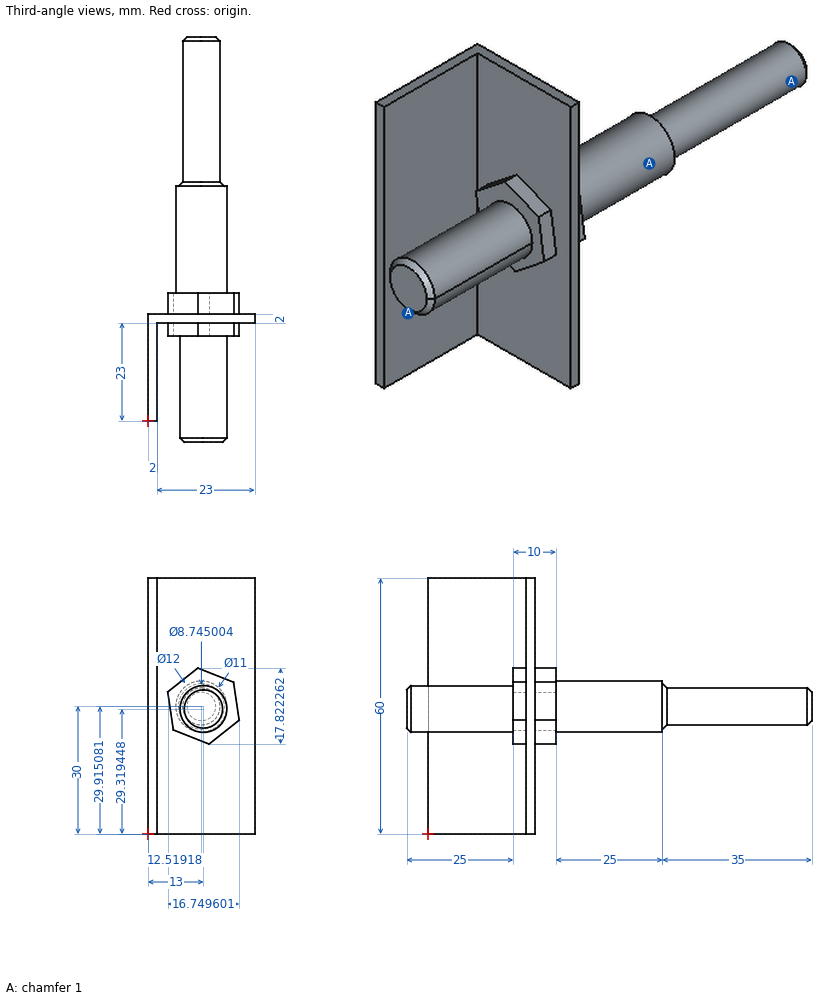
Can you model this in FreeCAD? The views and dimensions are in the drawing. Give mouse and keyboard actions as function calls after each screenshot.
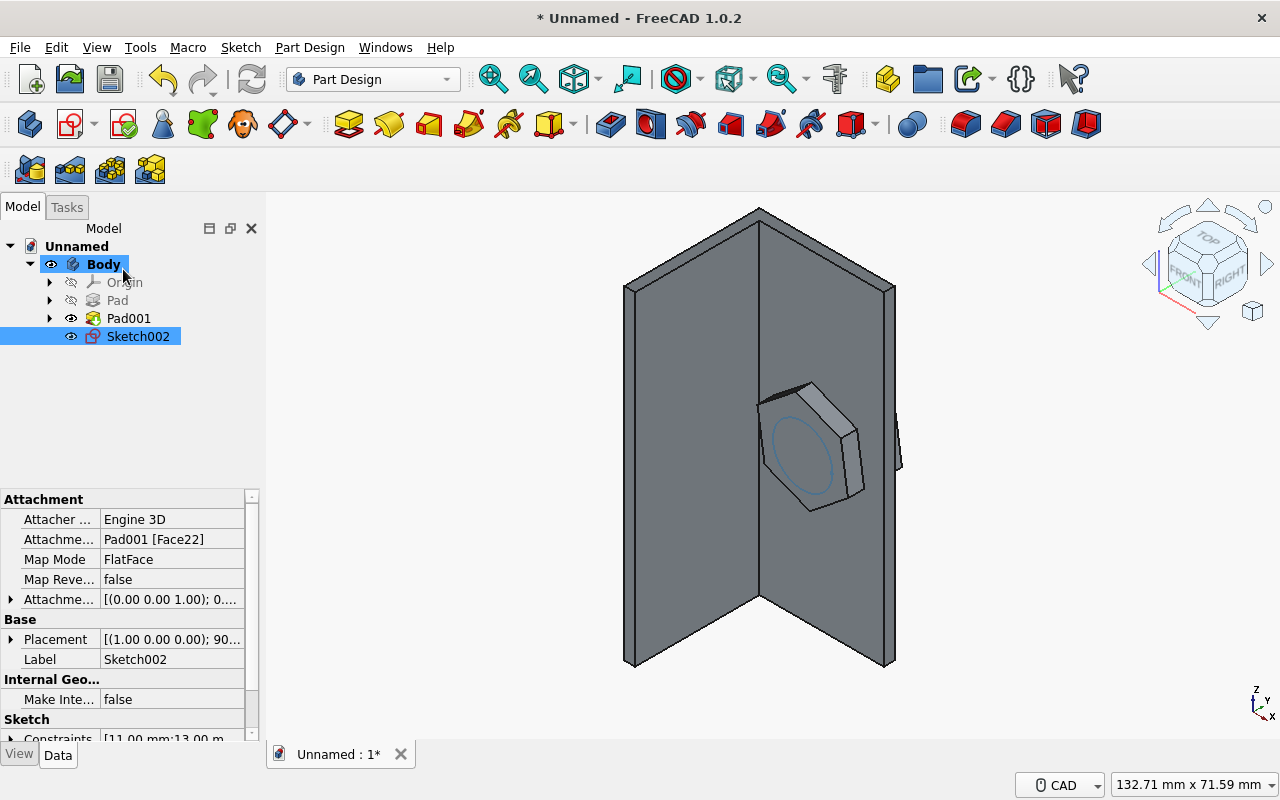
click(350, 124)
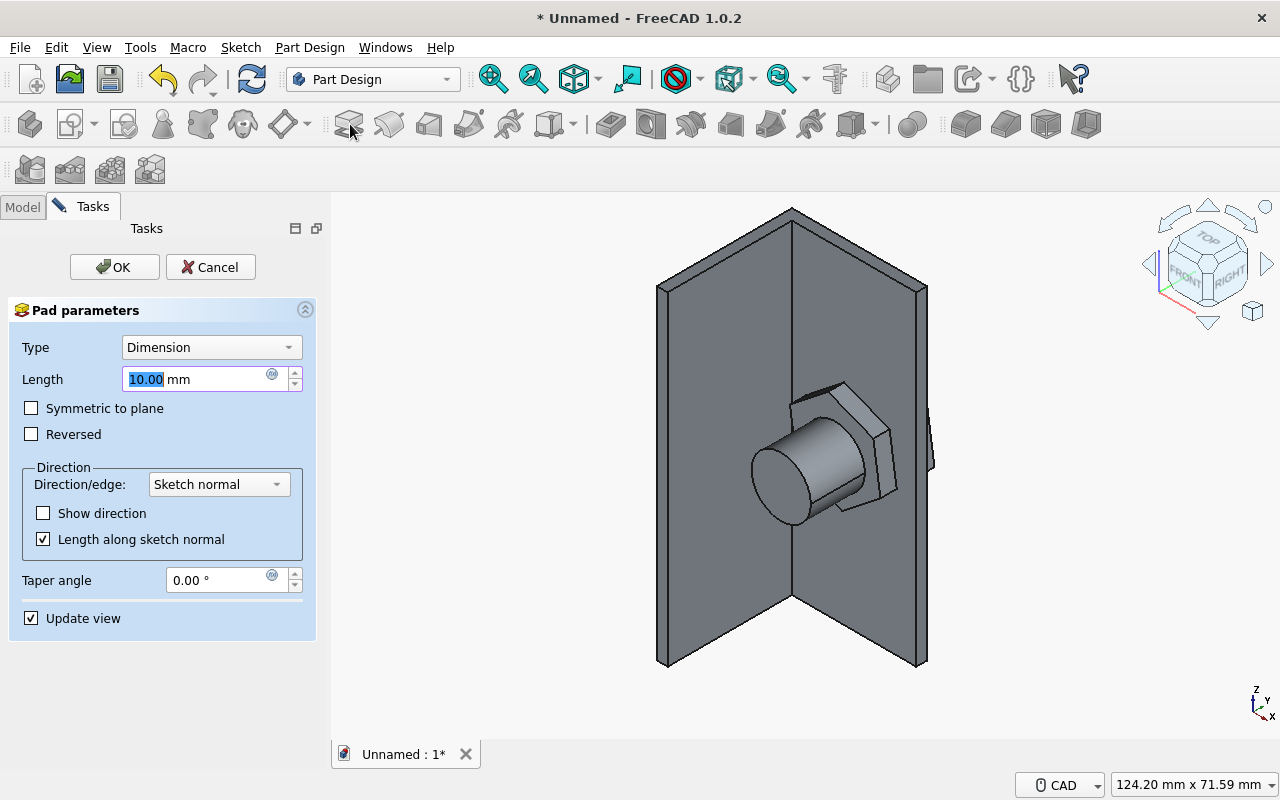
text(25)
key(Tab)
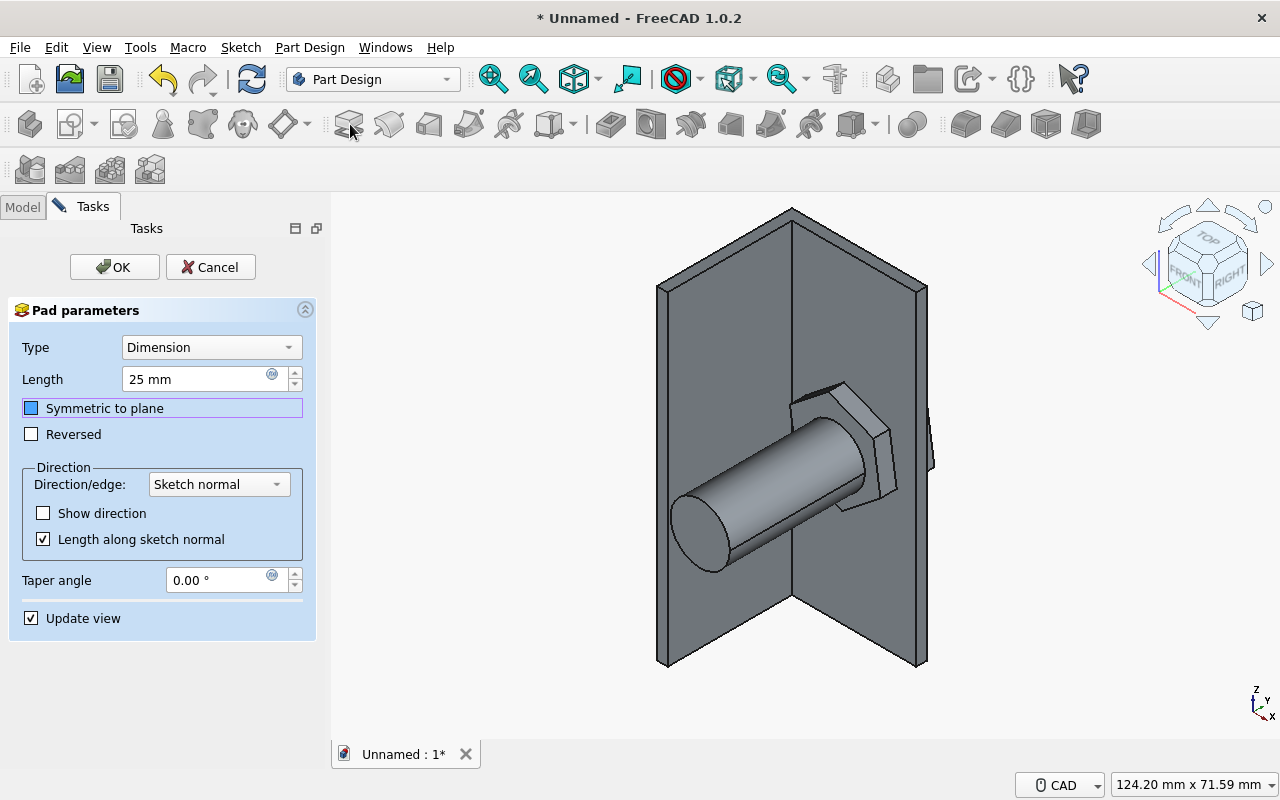
click(115, 267)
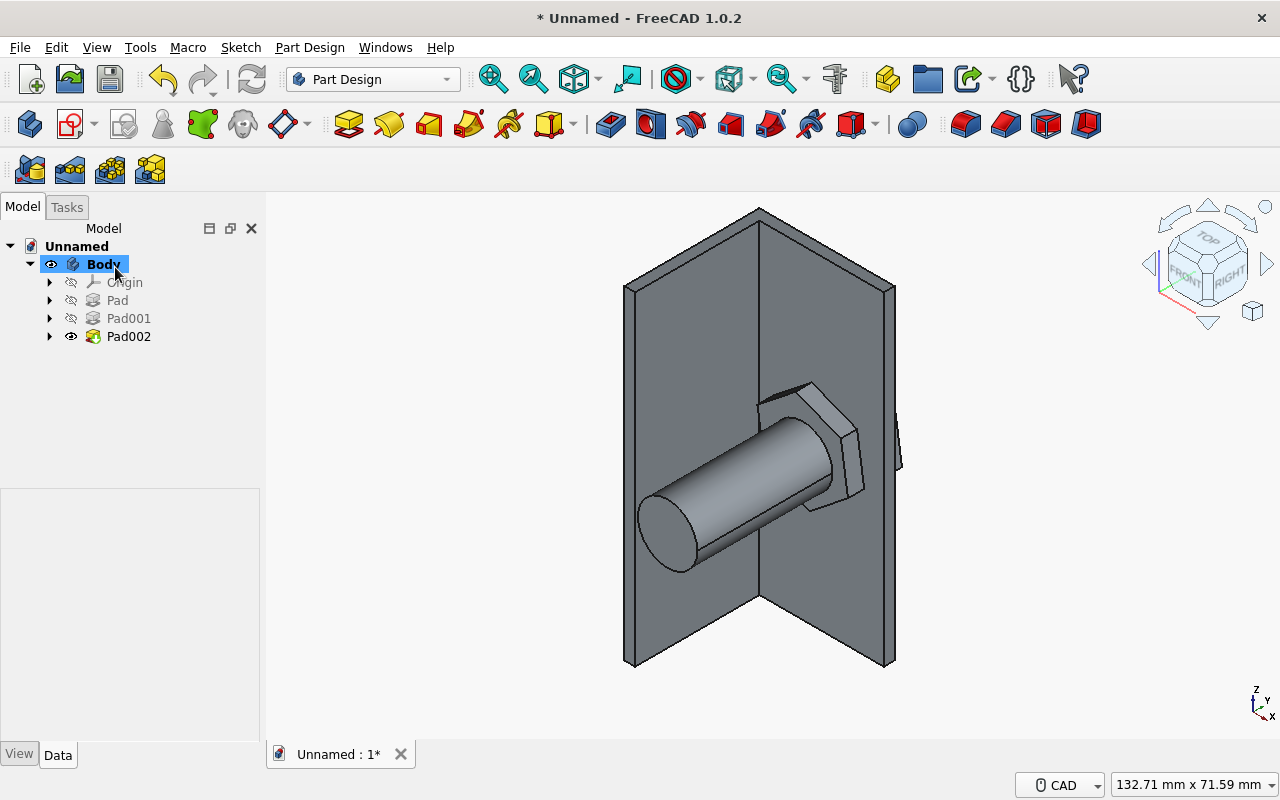
key(v)
key(f)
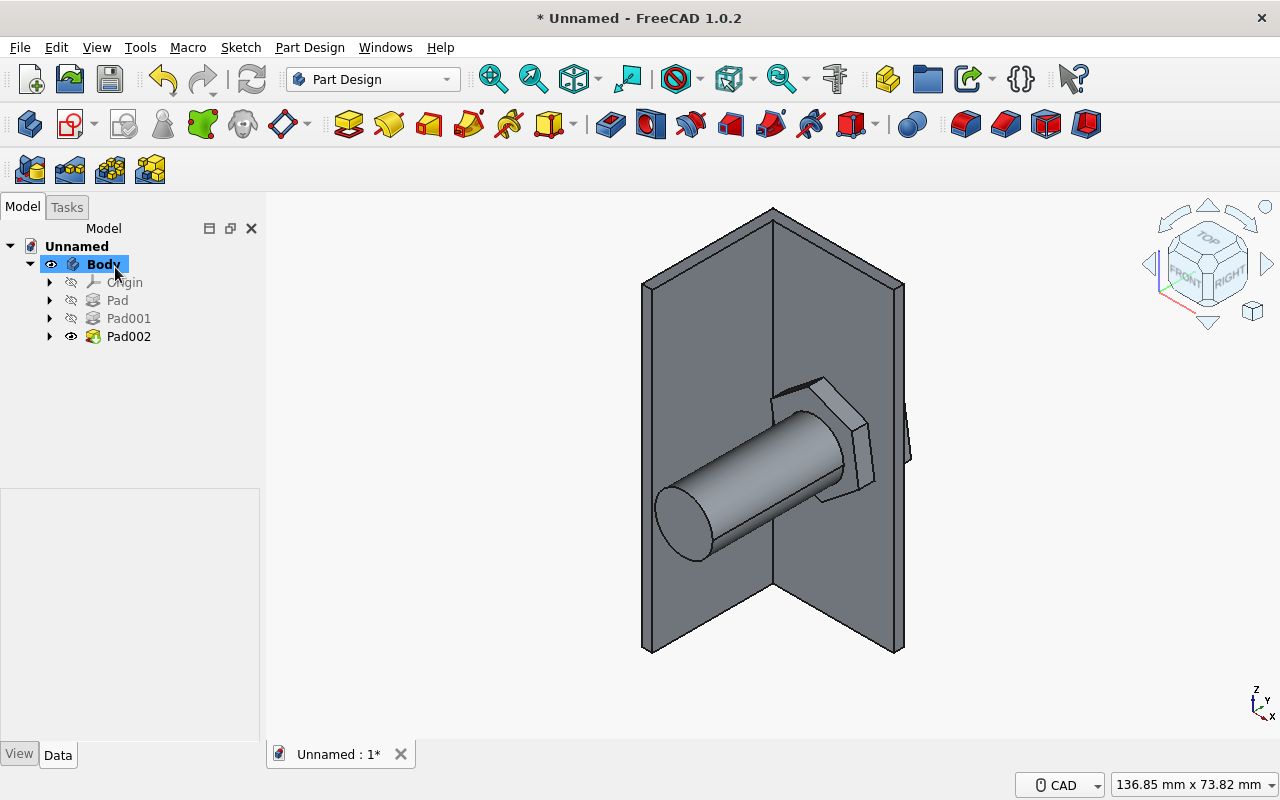
key(4)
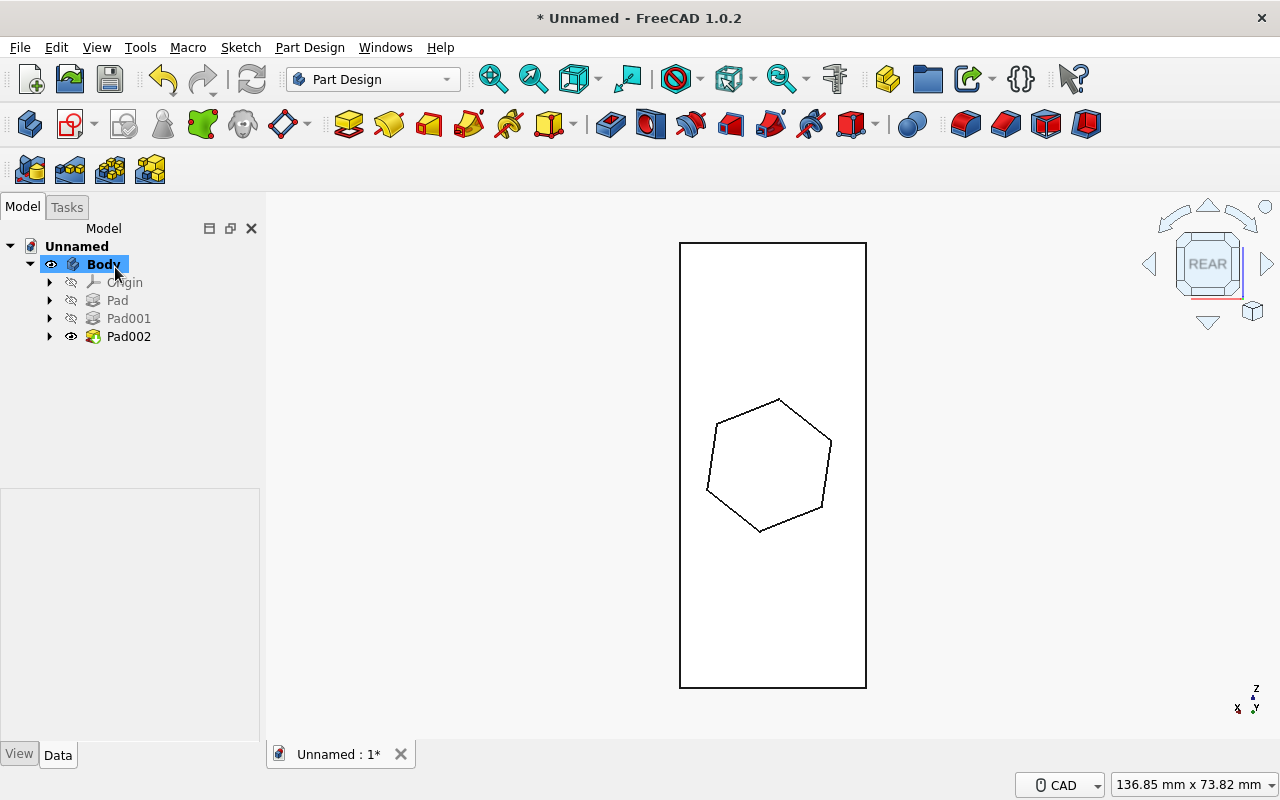
click(769, 465)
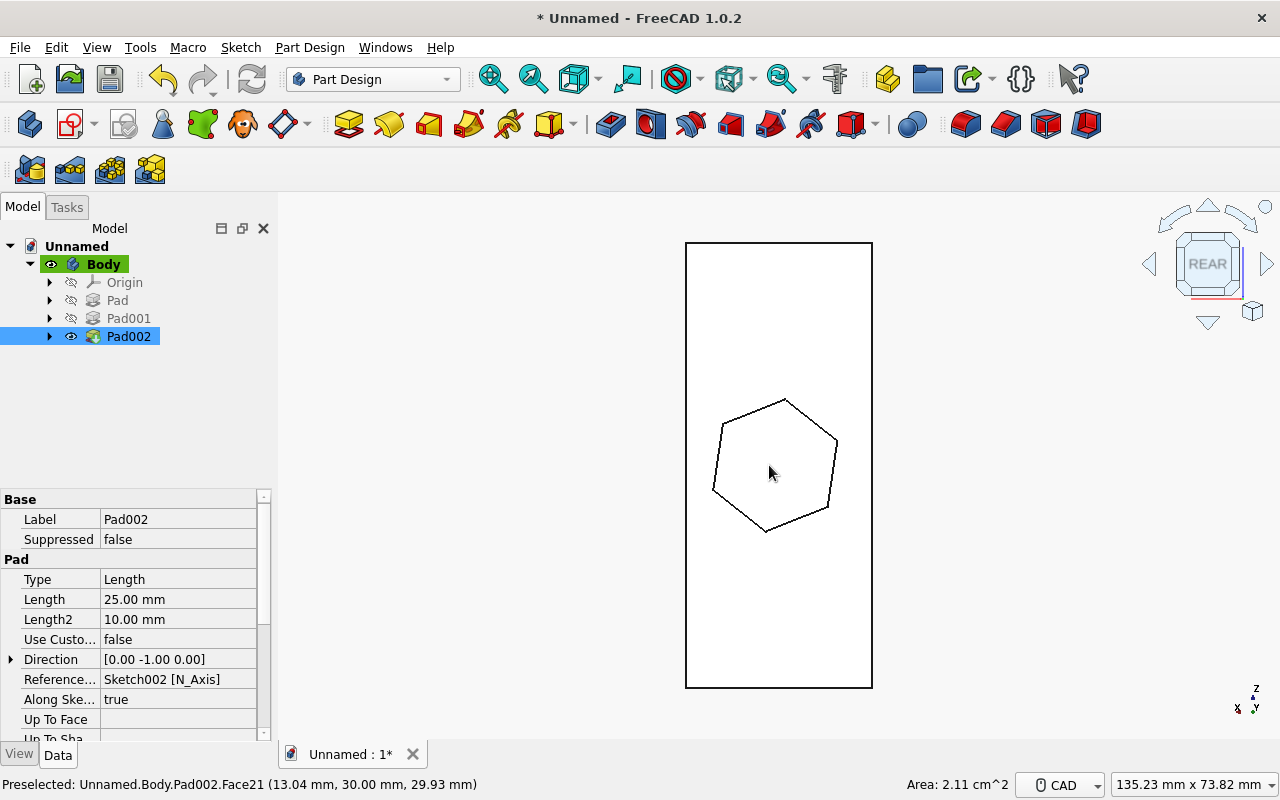
click(70, 124)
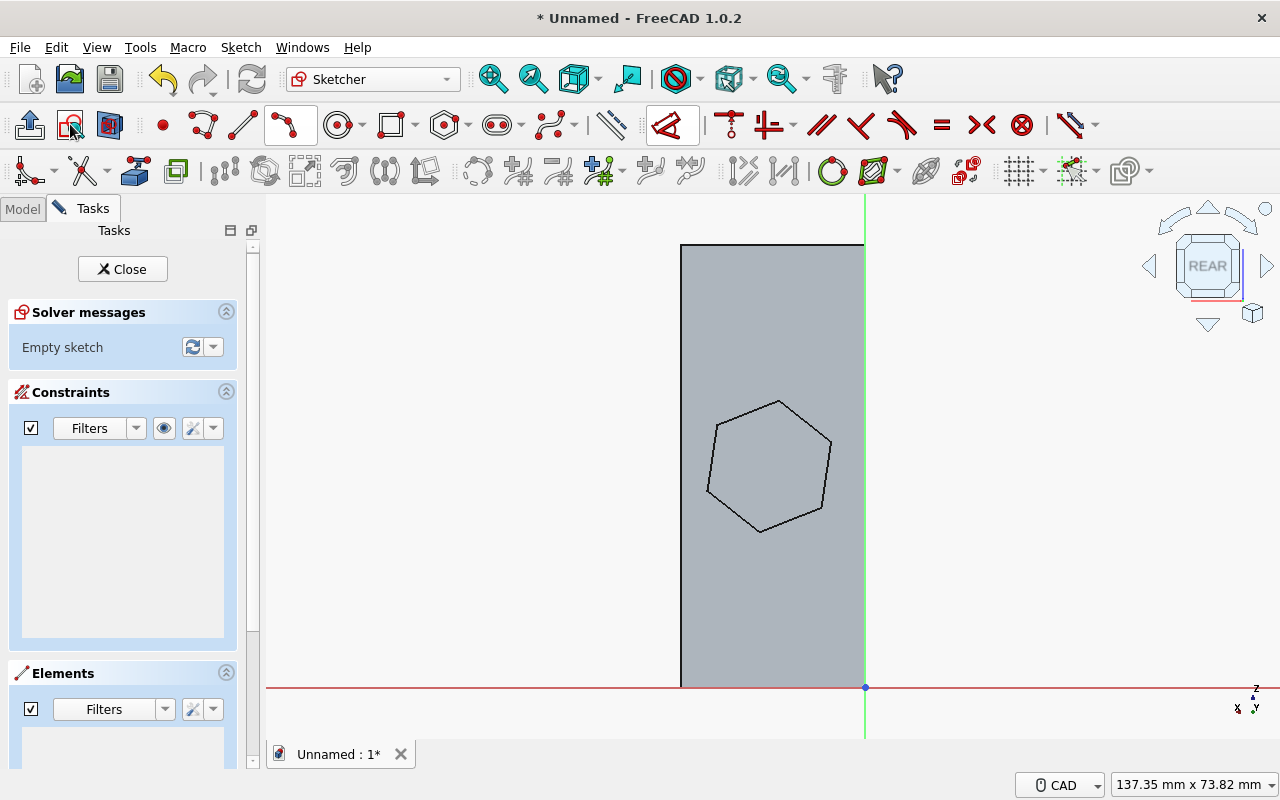
scroll(795, 467, up, 7)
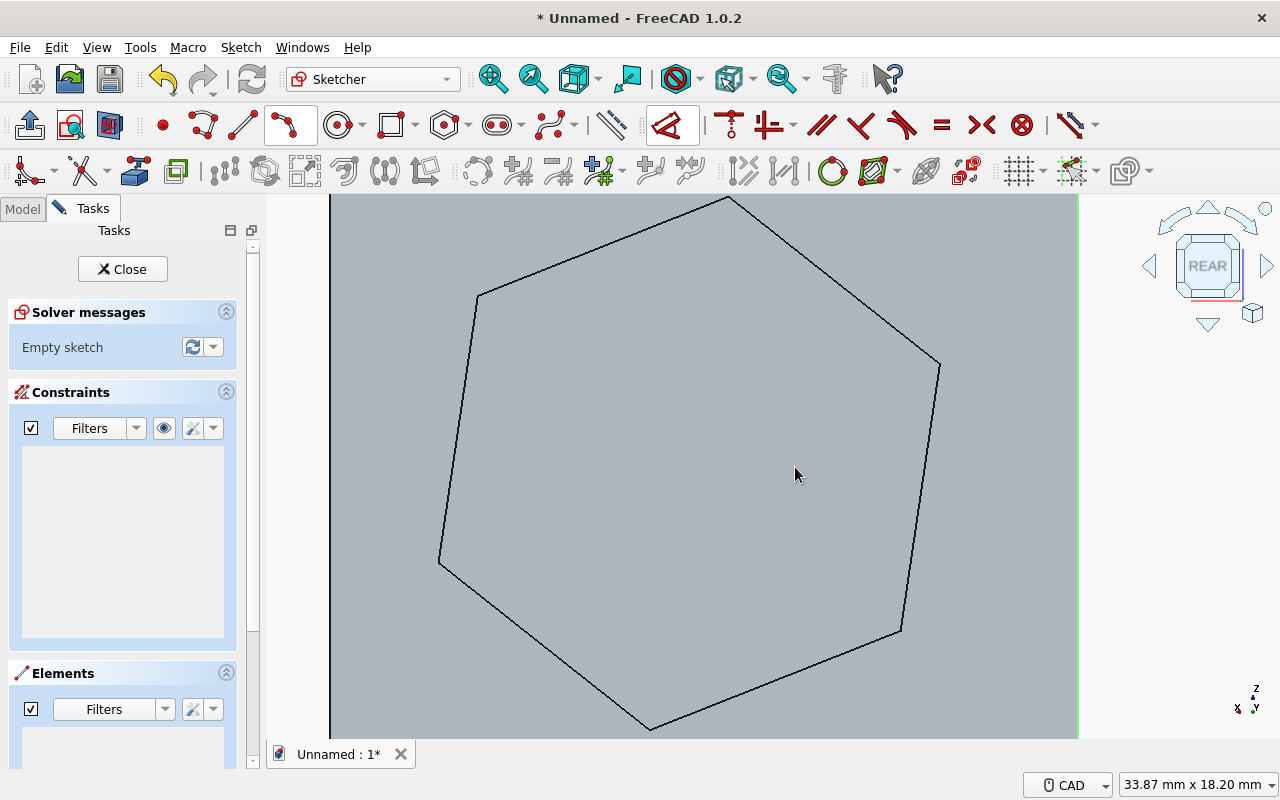
key(g)
key(c)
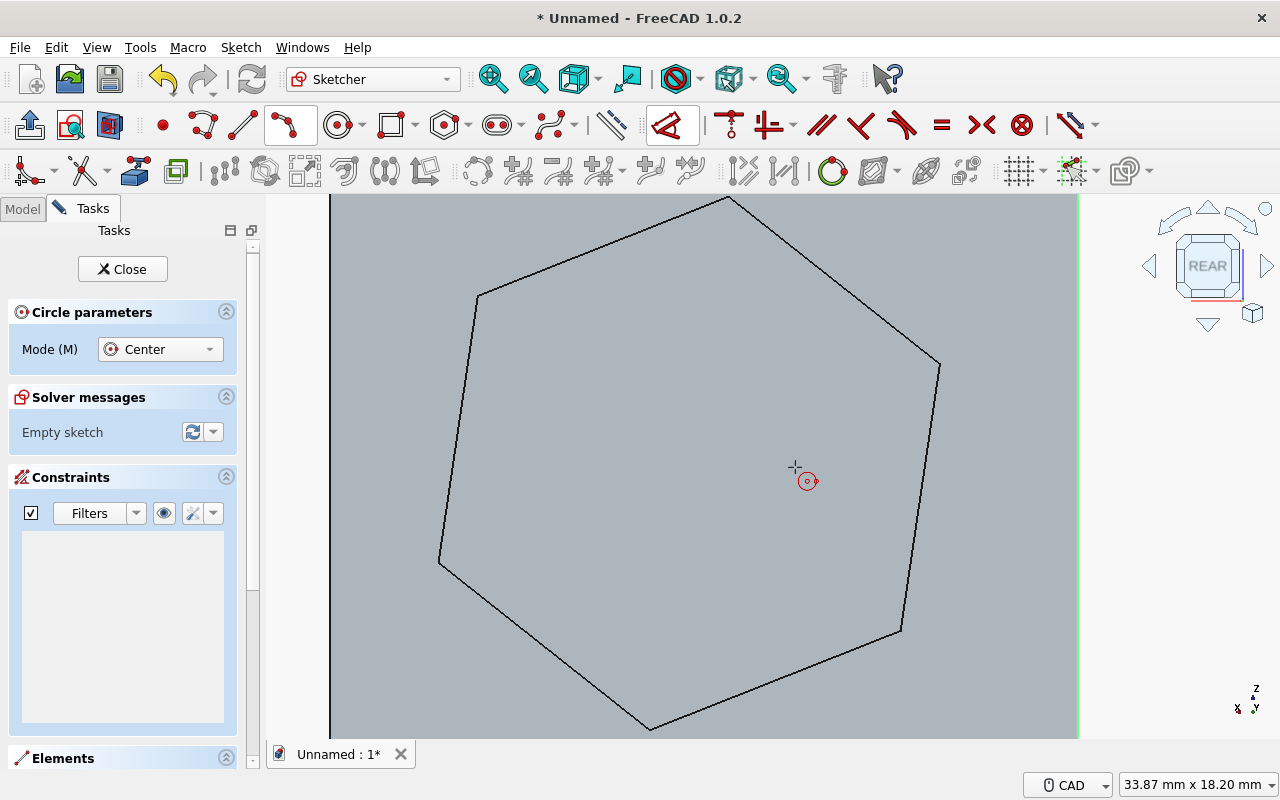
click(704, 466)
click(831, 339)
key(Escape)